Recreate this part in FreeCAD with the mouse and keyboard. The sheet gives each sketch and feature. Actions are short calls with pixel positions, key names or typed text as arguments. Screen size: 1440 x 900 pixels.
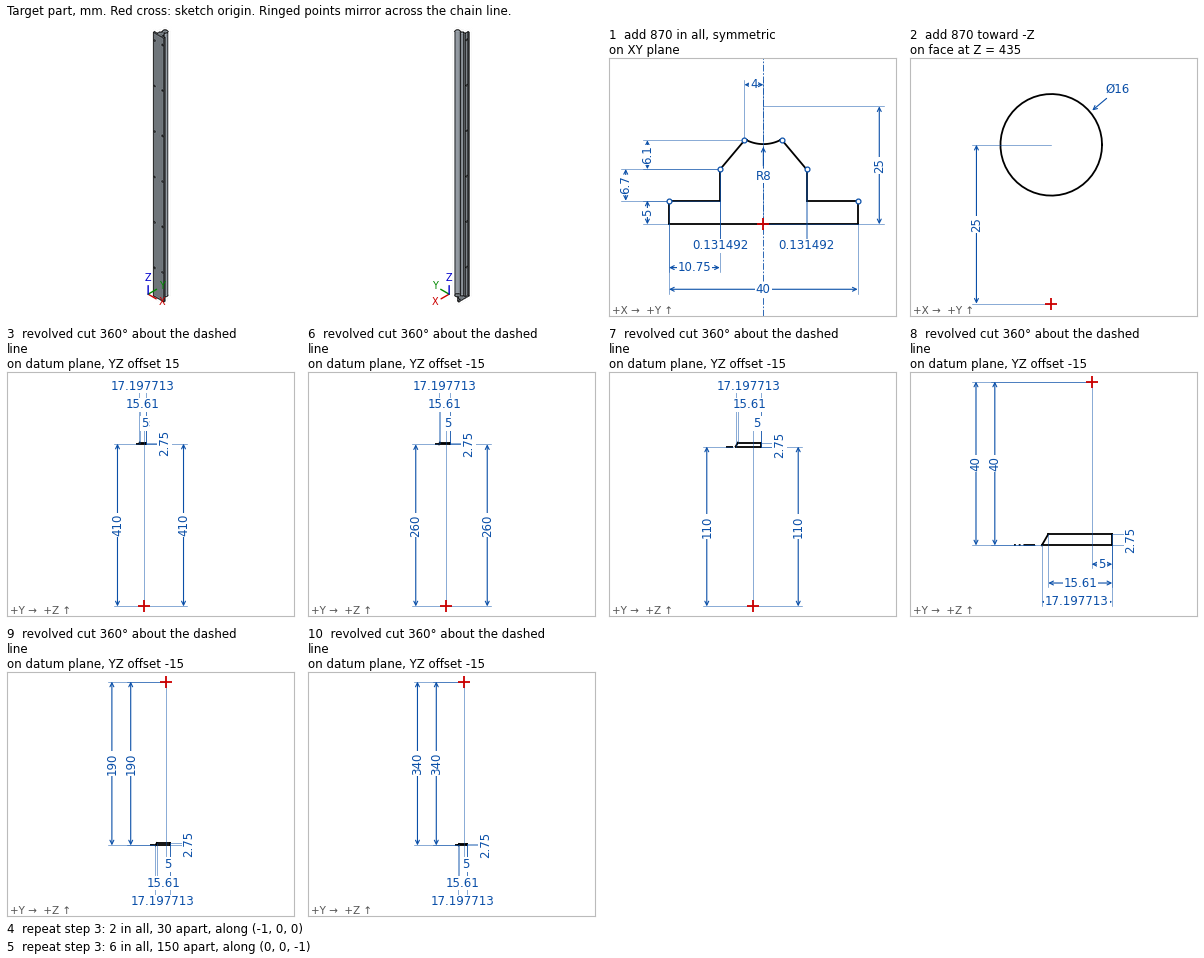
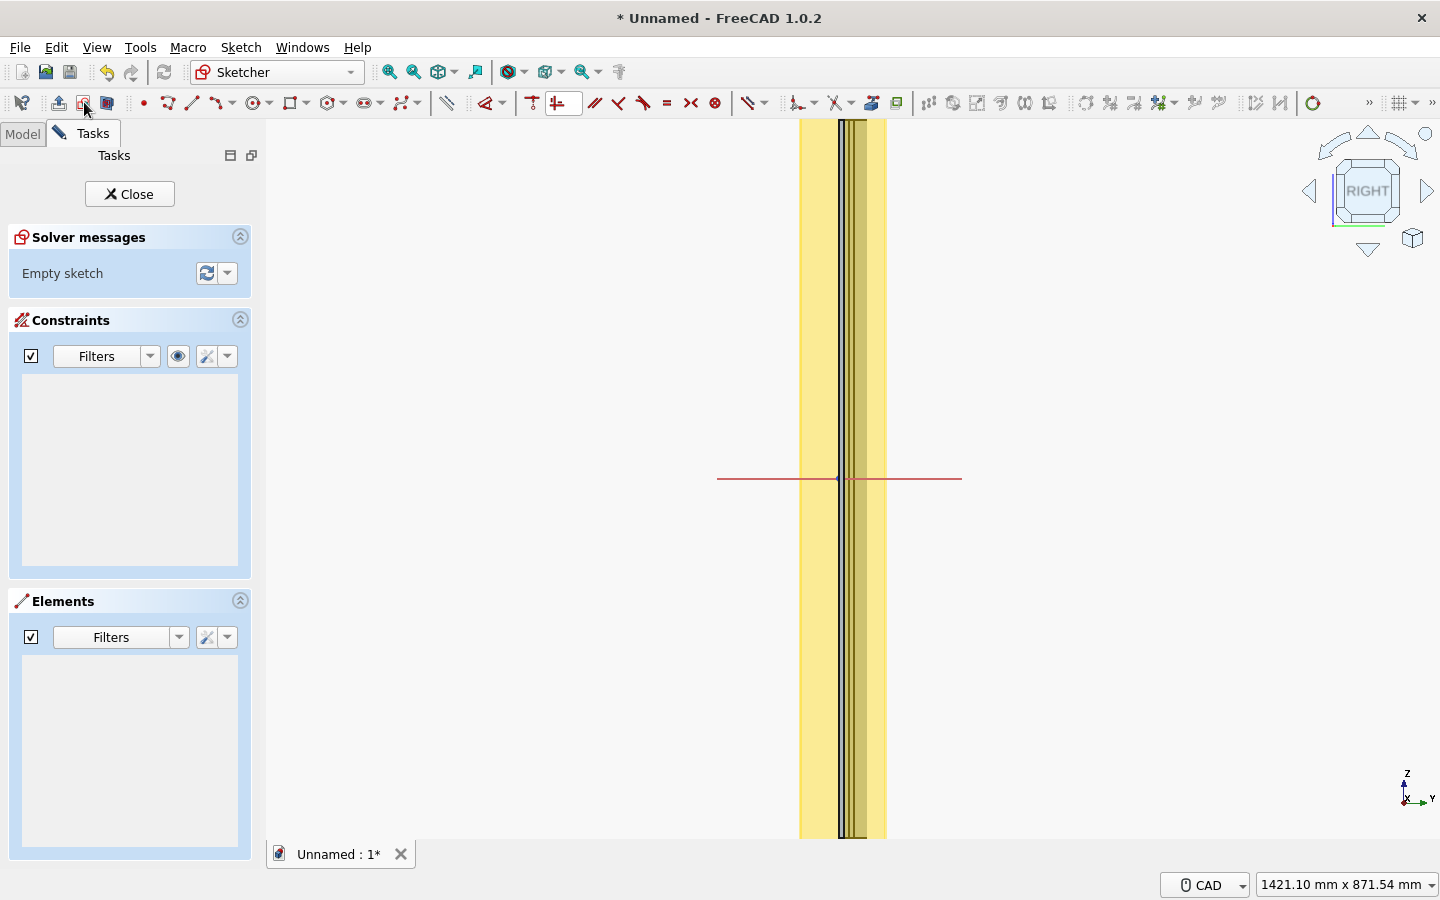
click(108, 104)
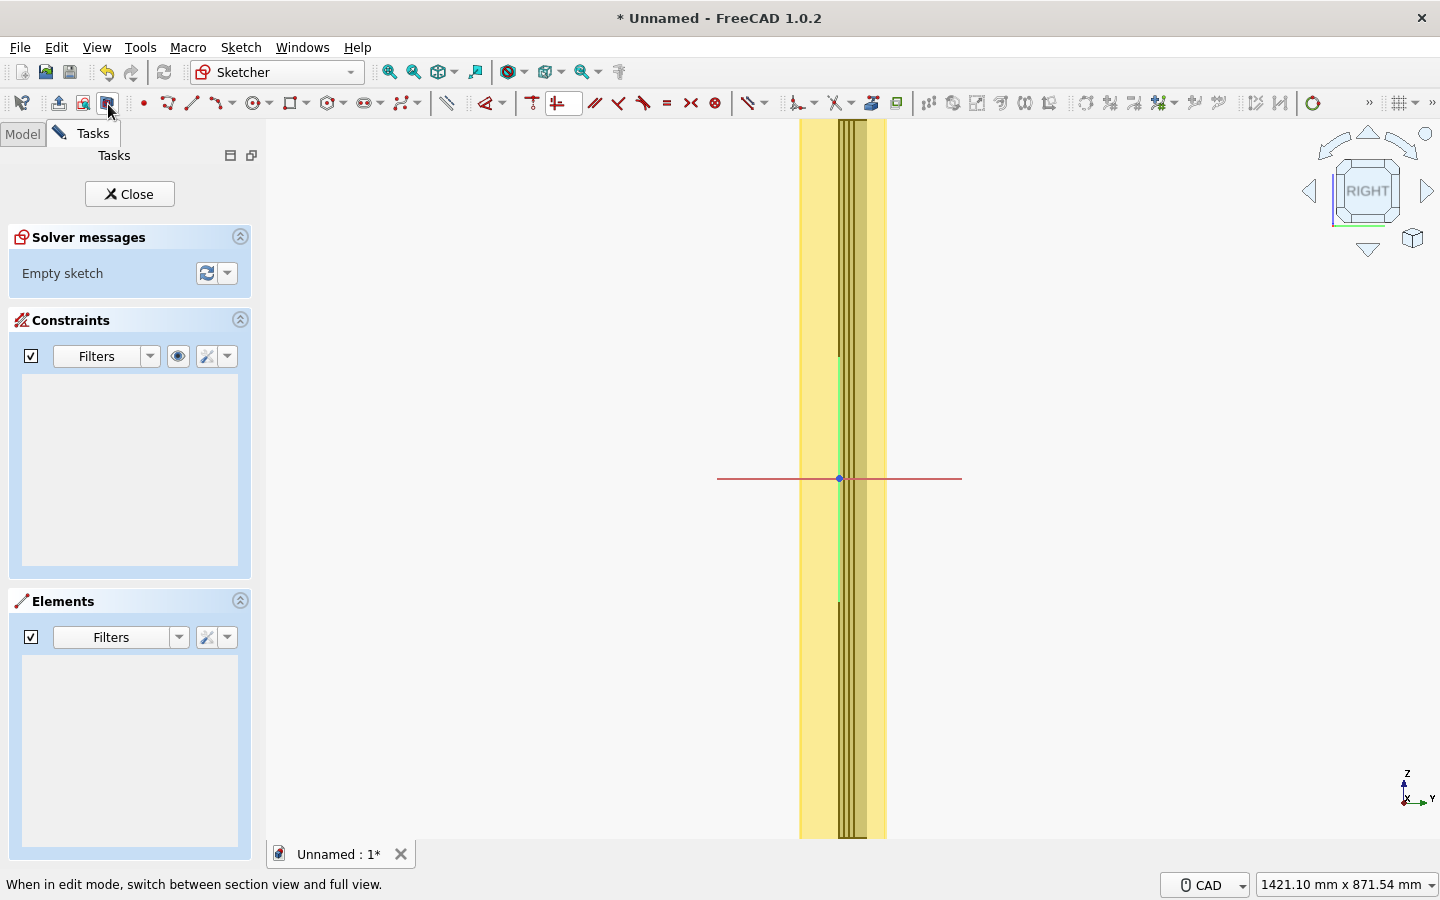
scroll(784, 479, down, 5)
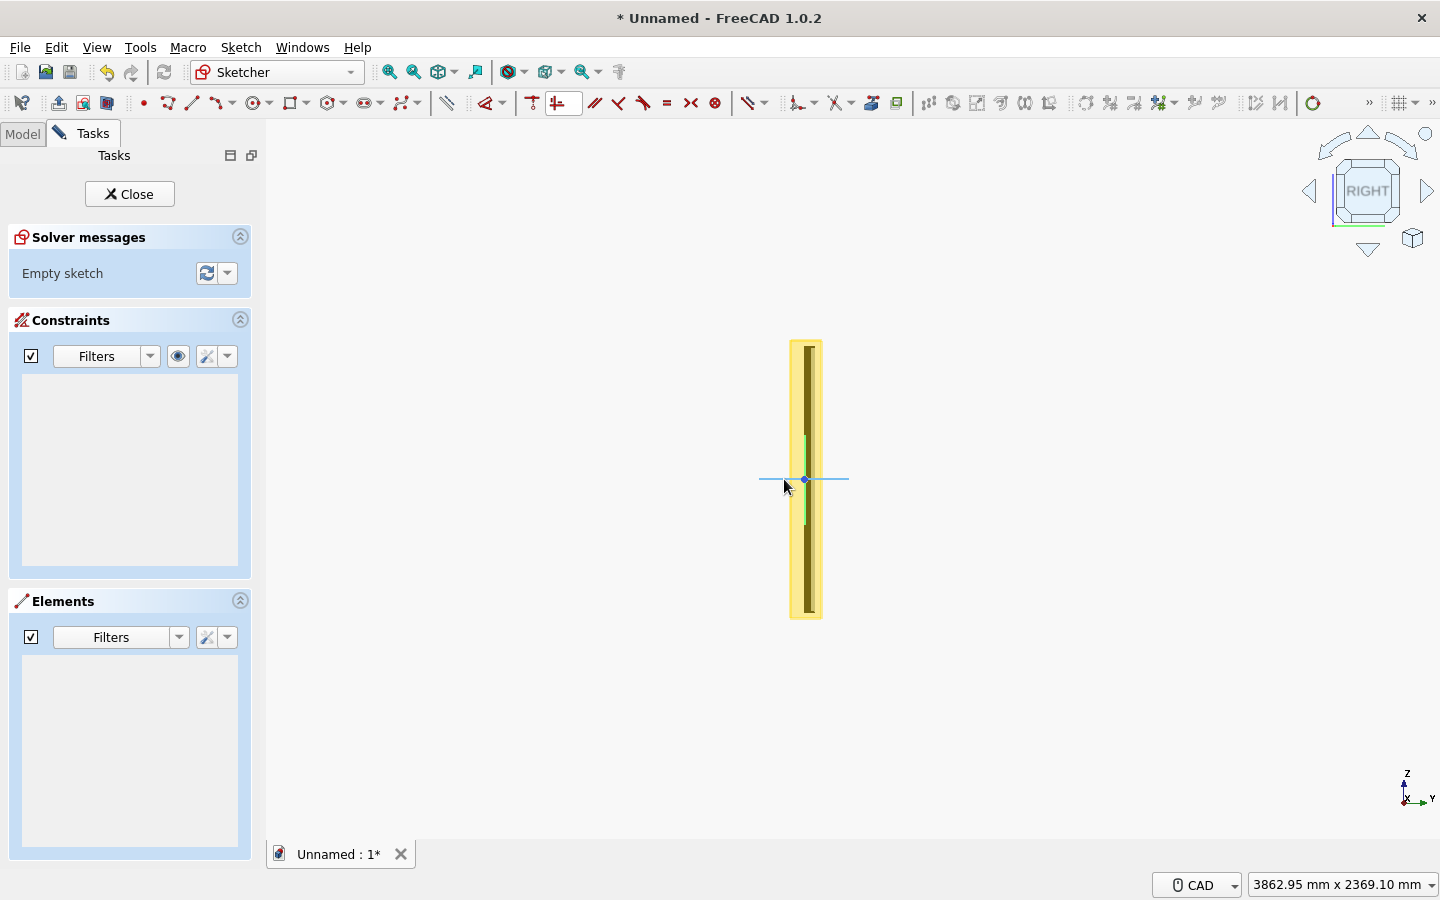
scroll(803, 348, up, 15)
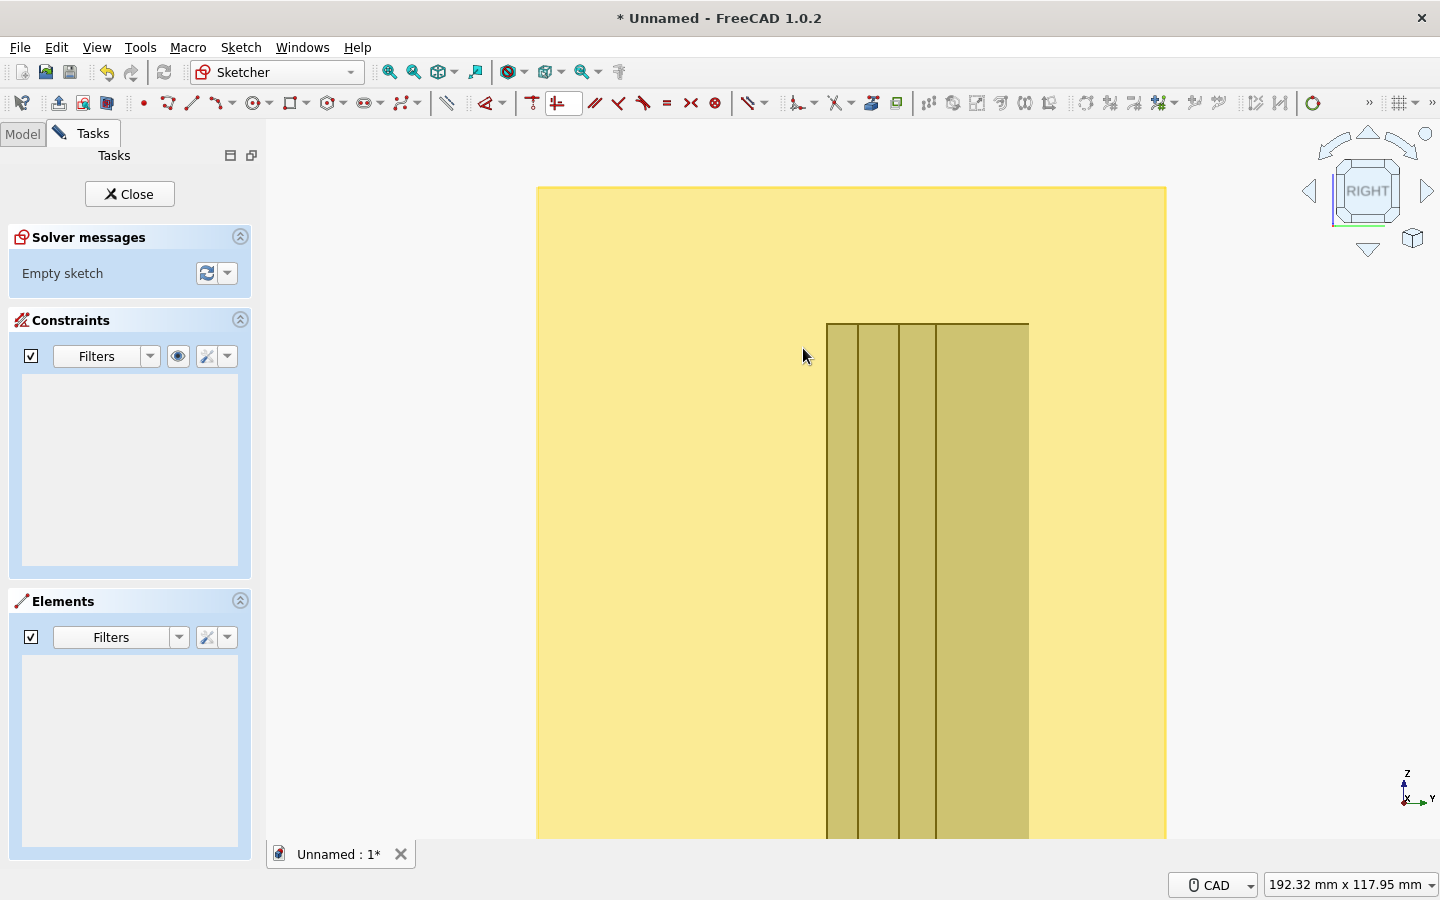
scroll(784, 466, up, 8)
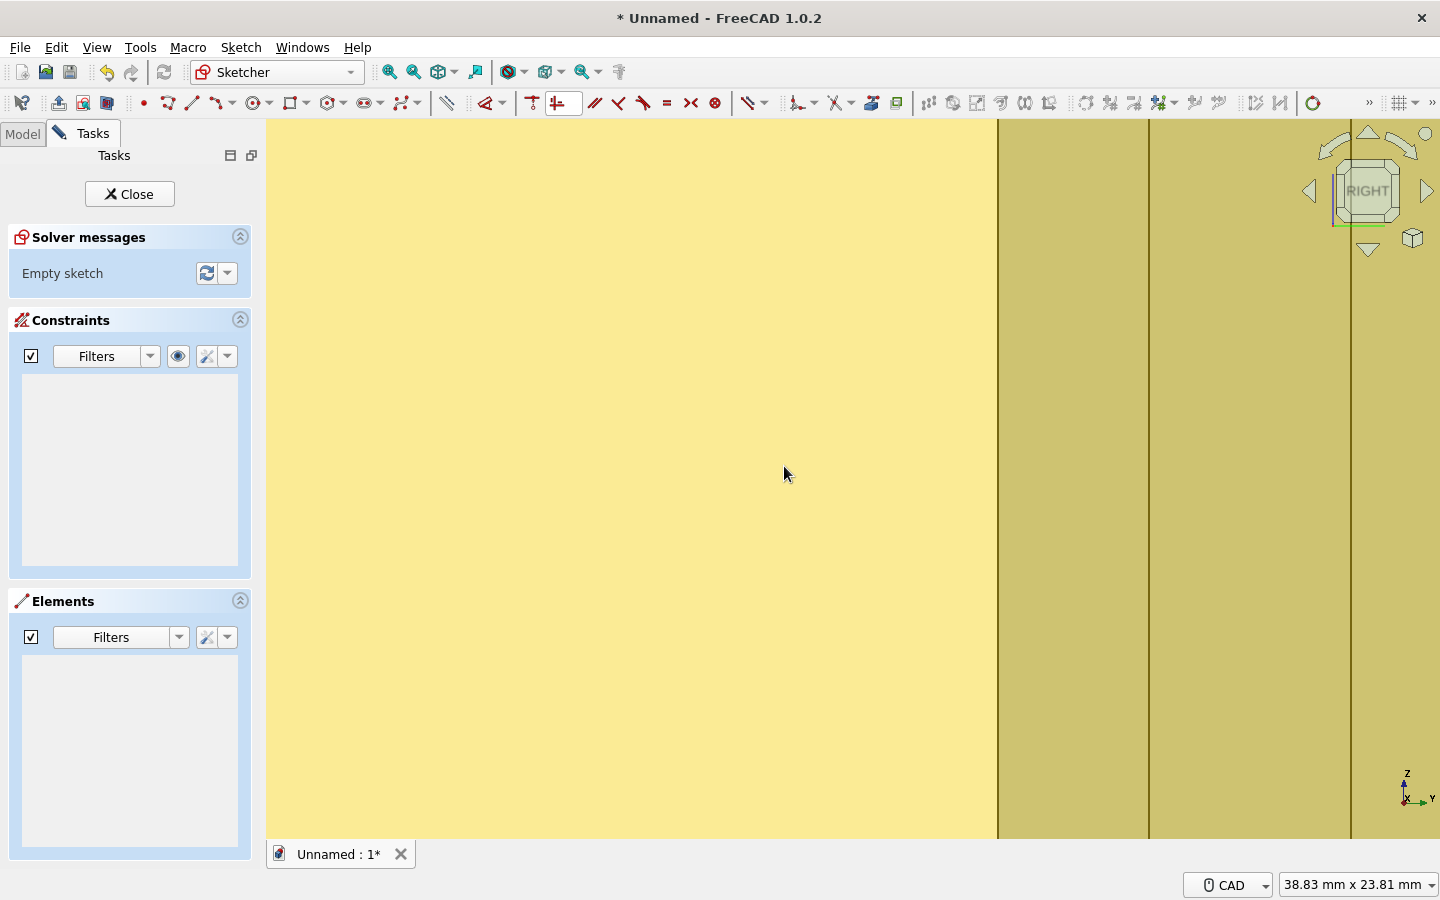
click(168, 104)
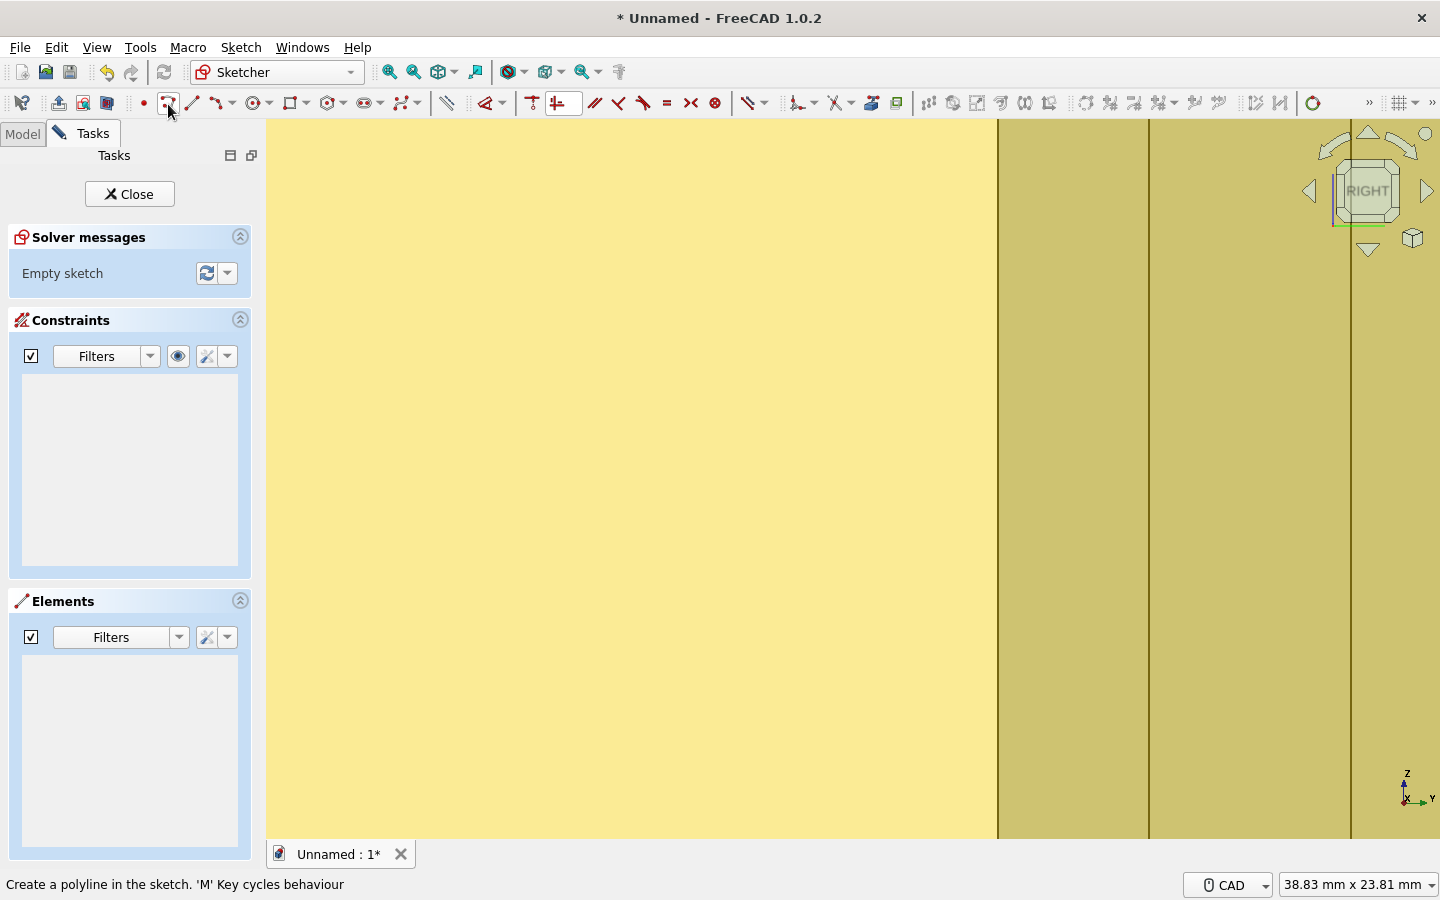
click(1149, 517)
click(1149, 434)
click(677, 434)
click(629, 517)
click(1149, 518)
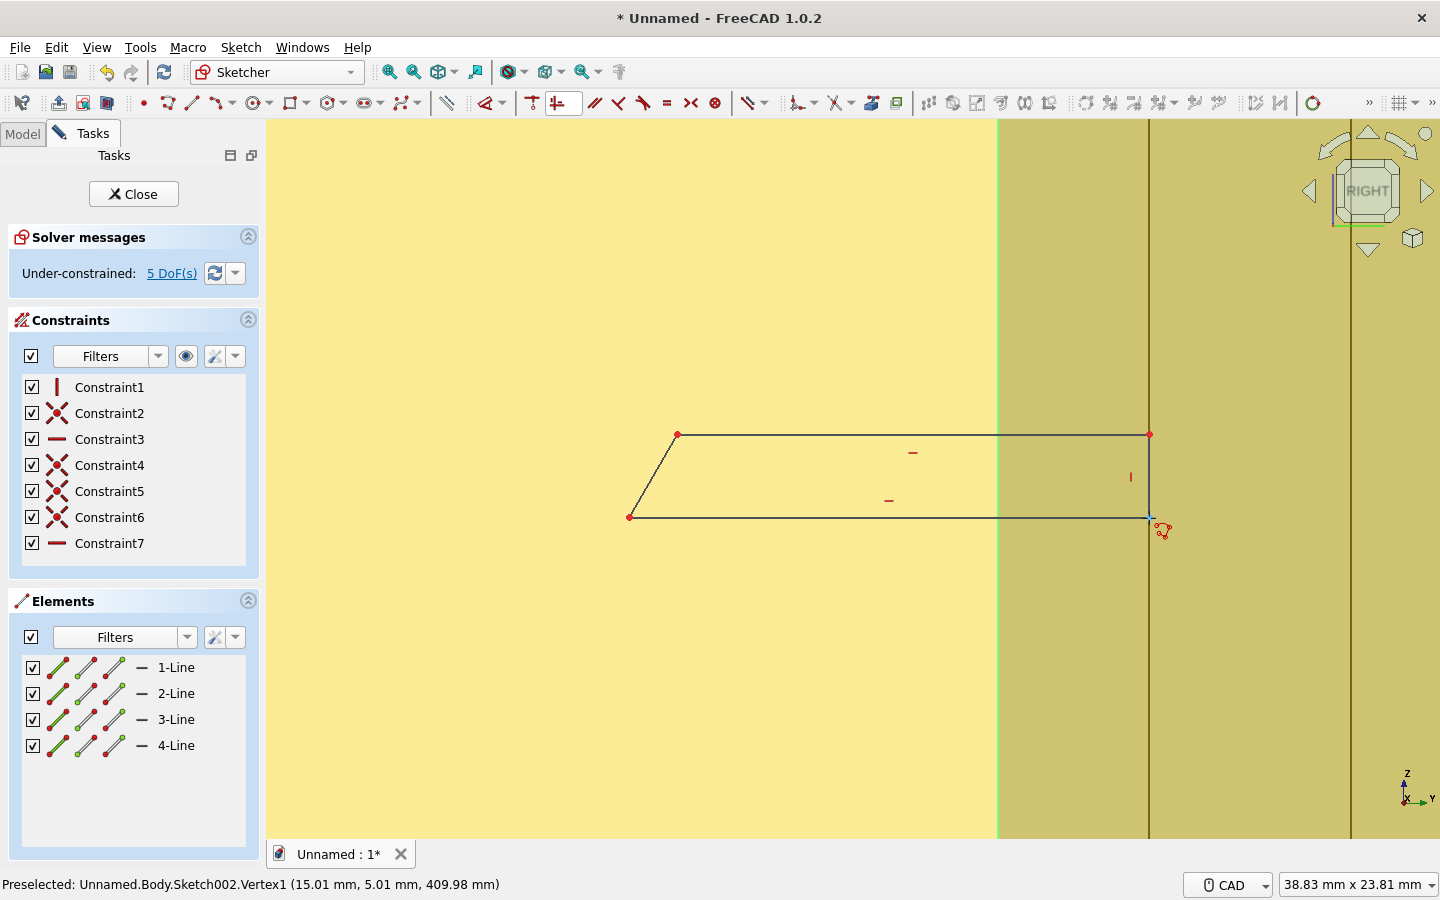
key(g)
key(l)